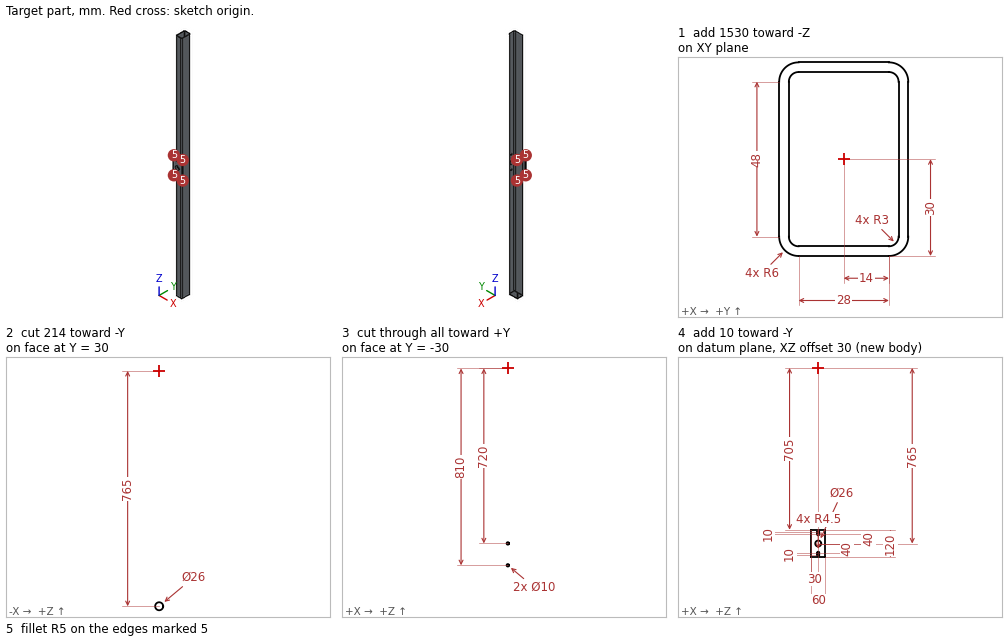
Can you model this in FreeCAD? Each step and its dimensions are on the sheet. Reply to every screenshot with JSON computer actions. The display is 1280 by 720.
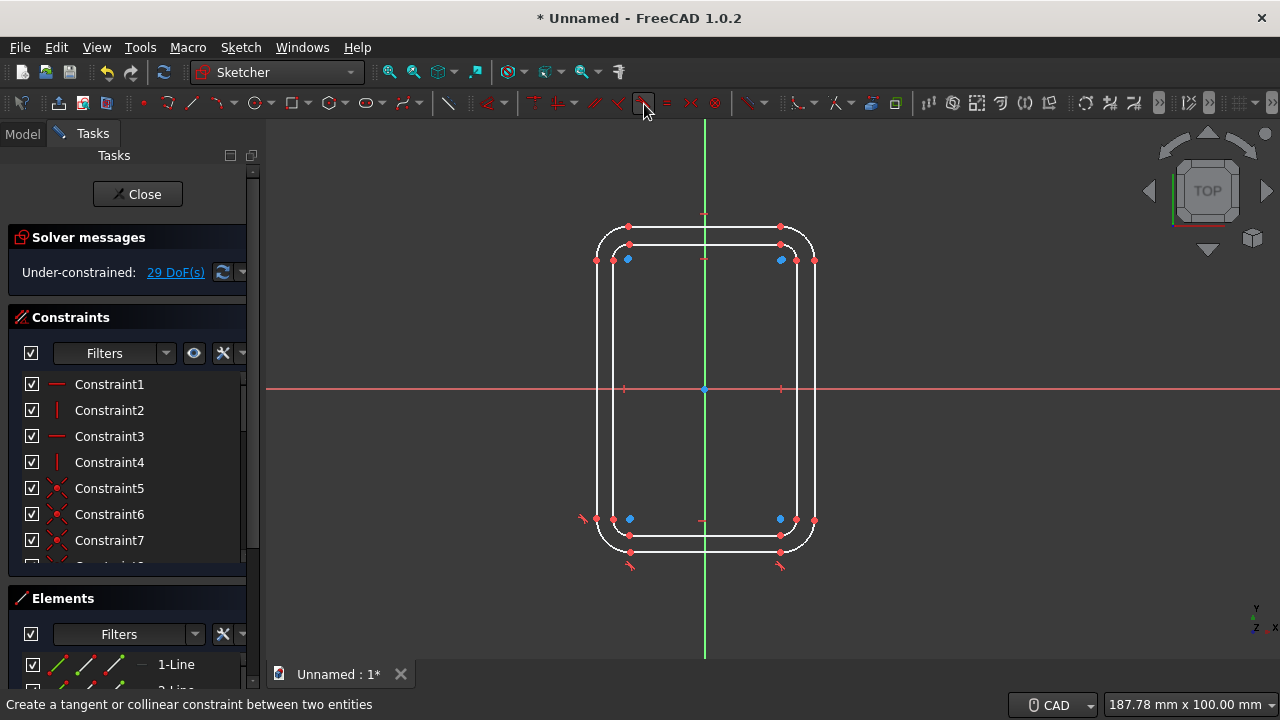
{"action": "left_click", "coordinate": [597, 441]}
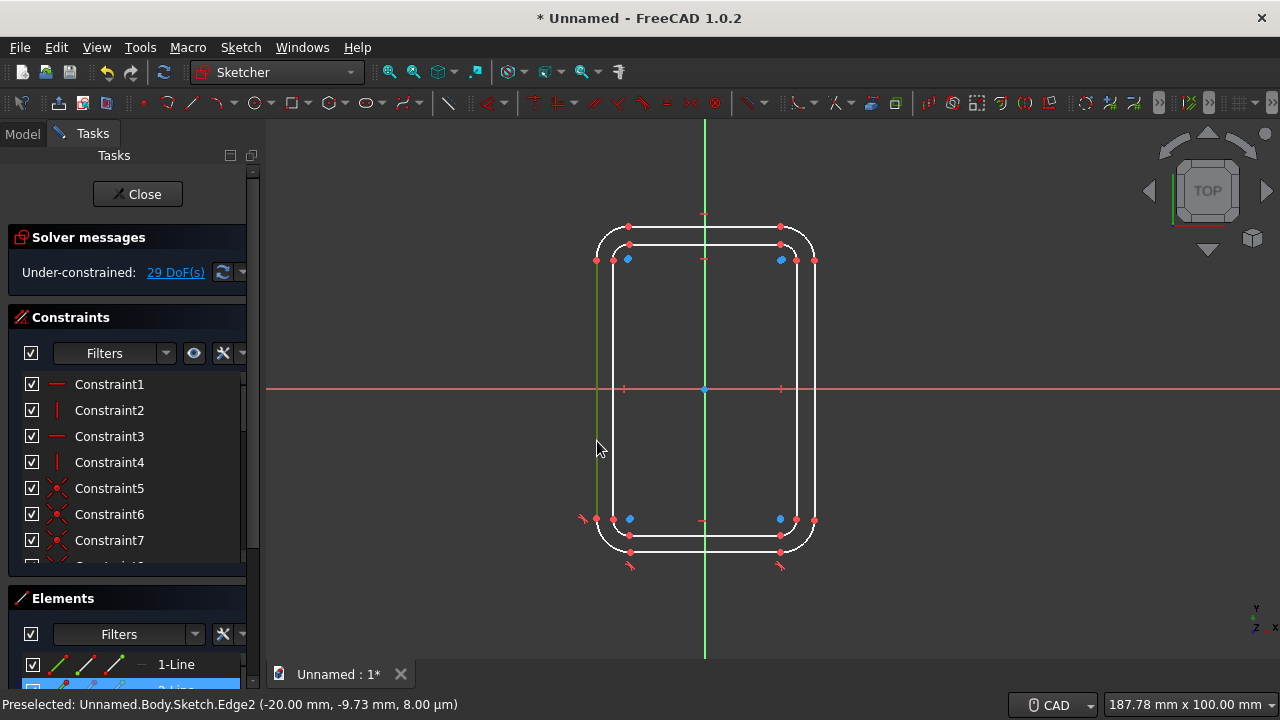
{"action": "left_click", "coordinate": [614, 230]}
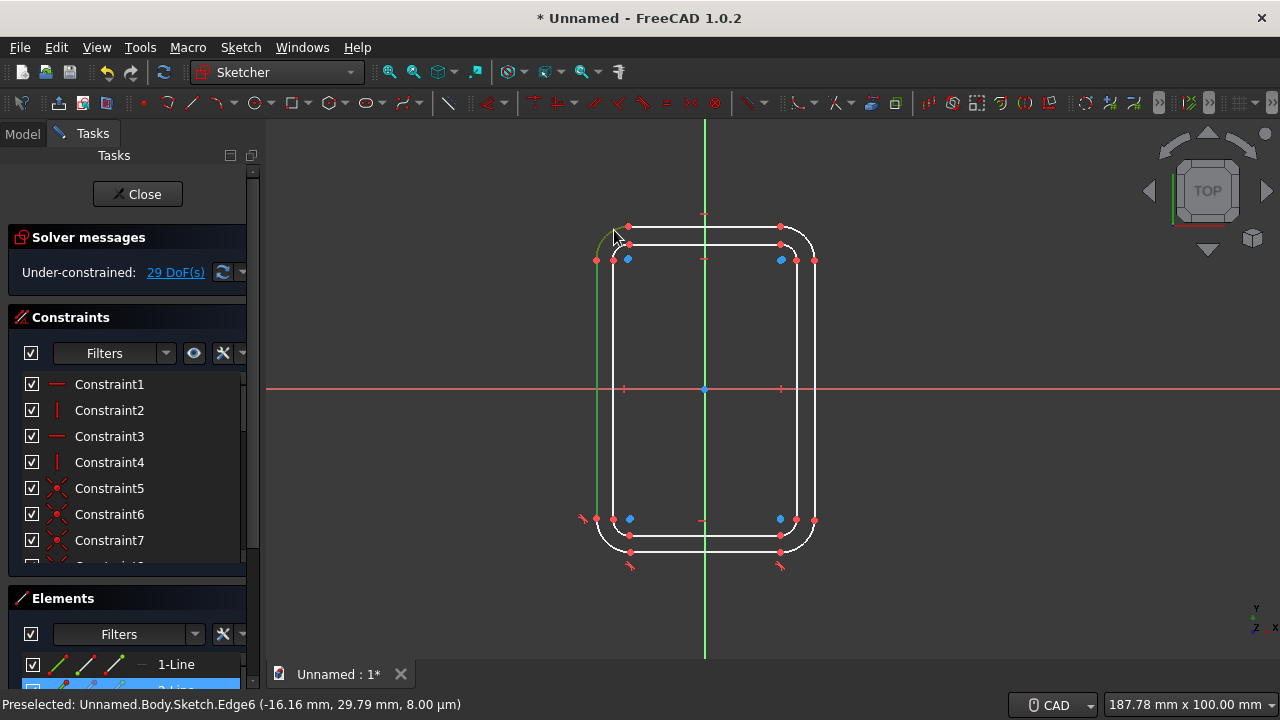
{"action": "left_click", "coordinate": [644, 104]}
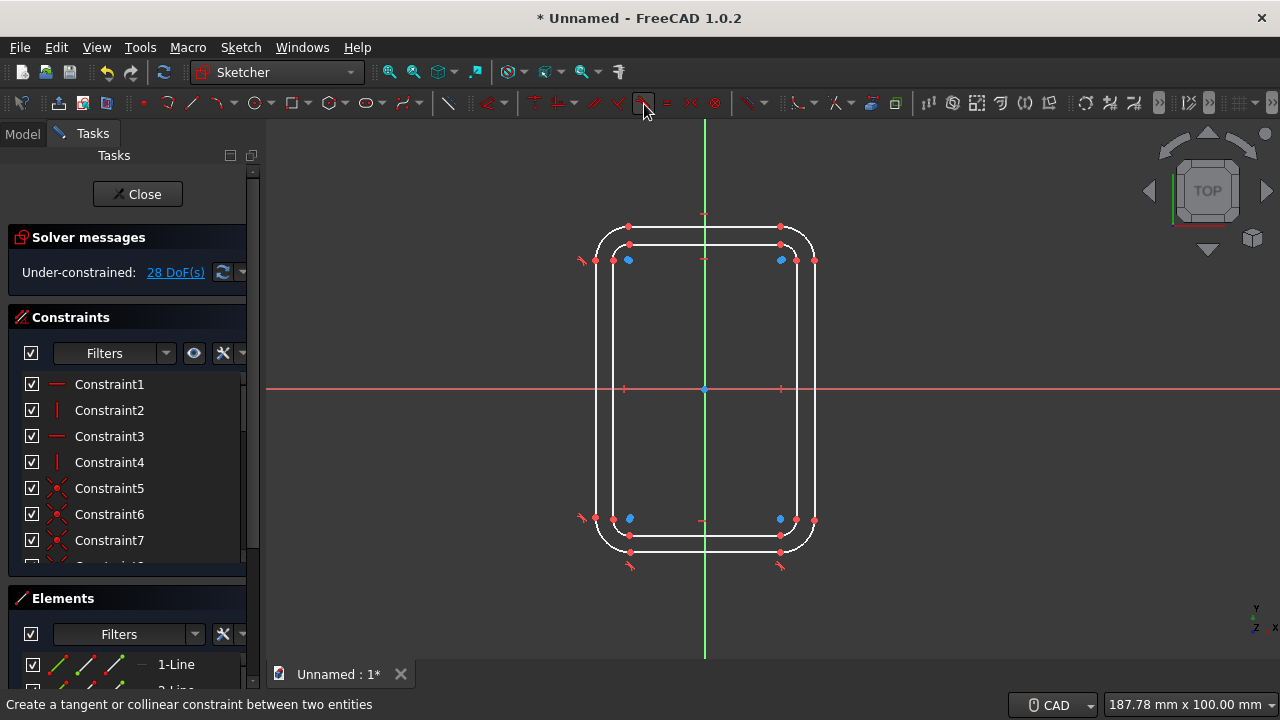
{"action": "left_click", "coordinate": [674, 227]}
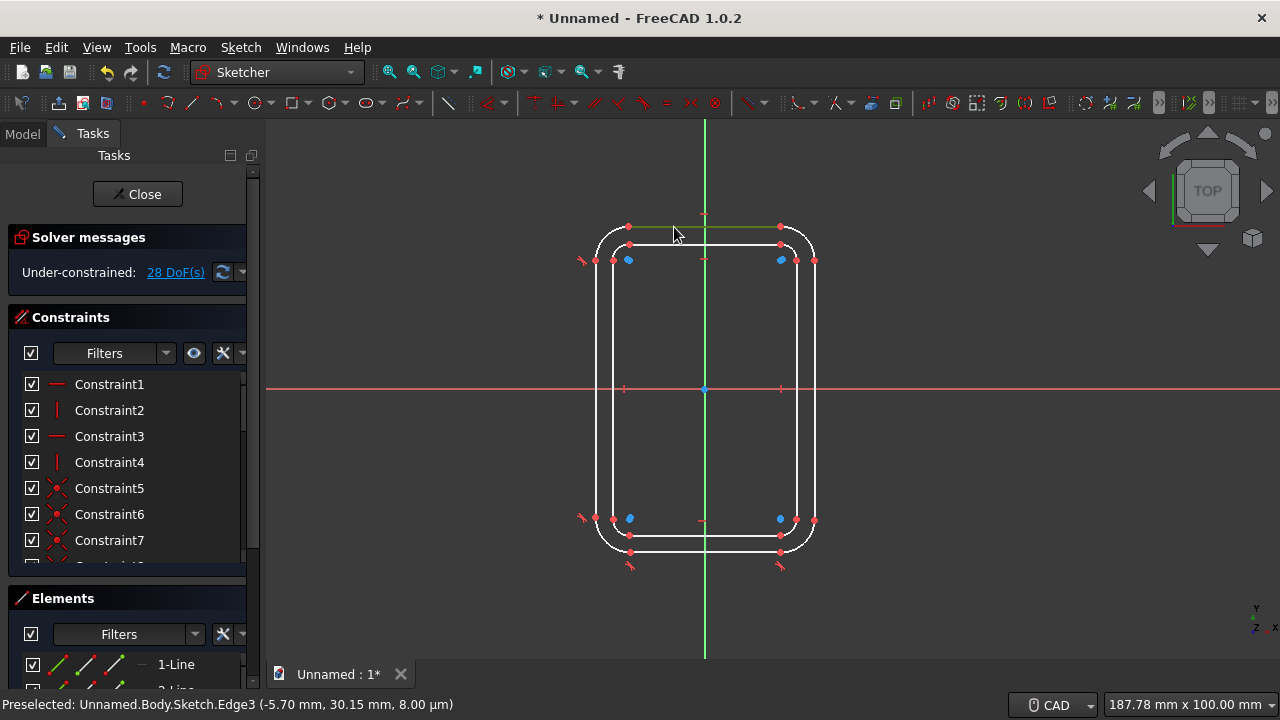
{"action": "left_click", "coordinate": [614, 231]}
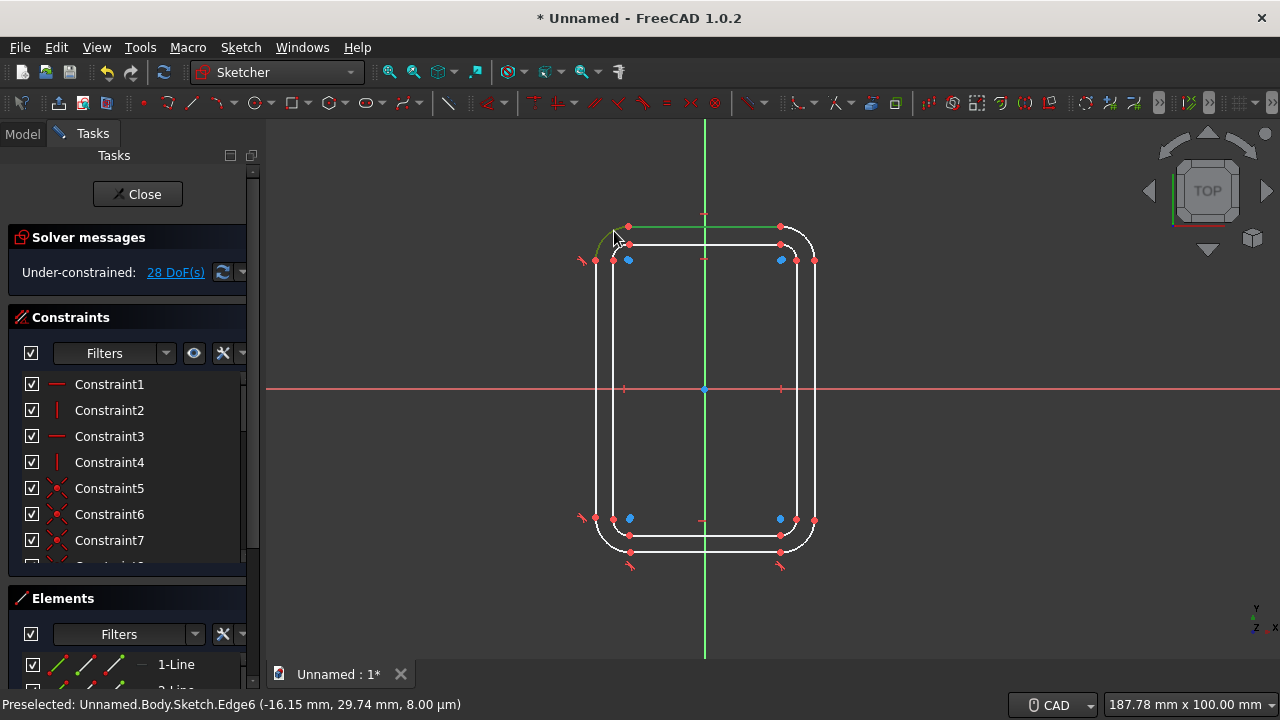
{"action": "left_click", "coordinate": [644, 104]}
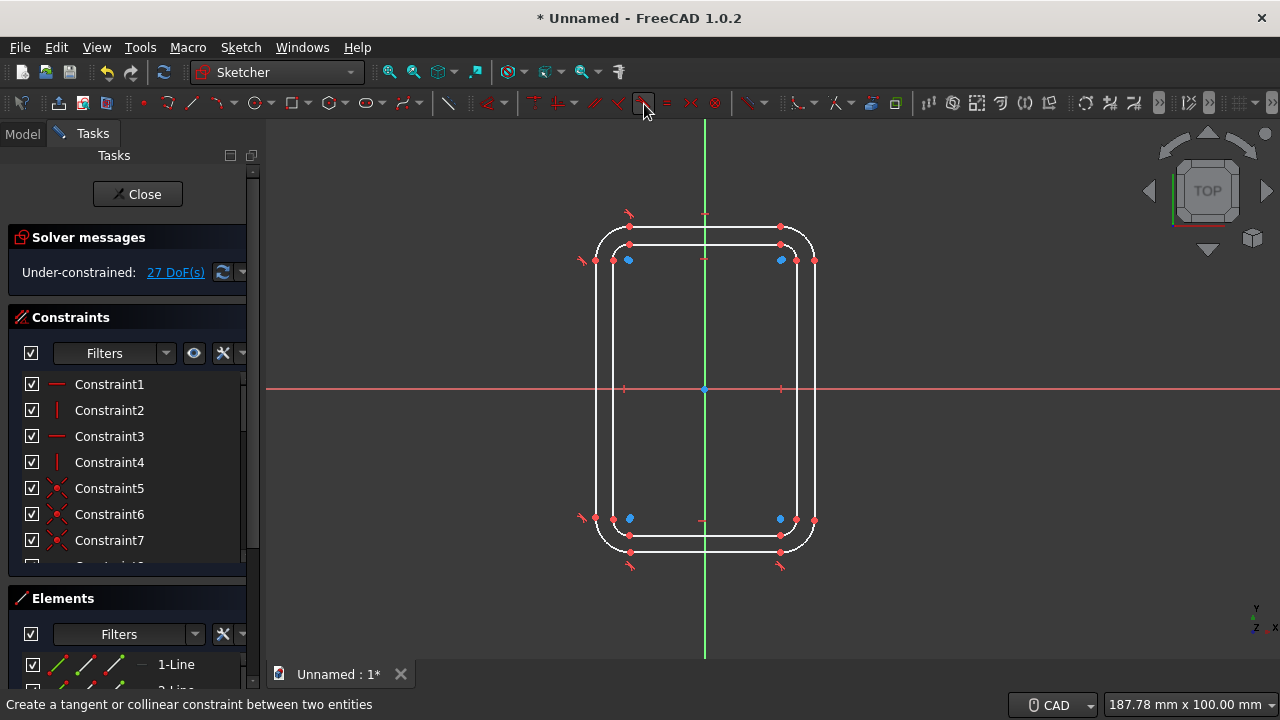
{"action": "left_click", "coordinate": [675, 227]}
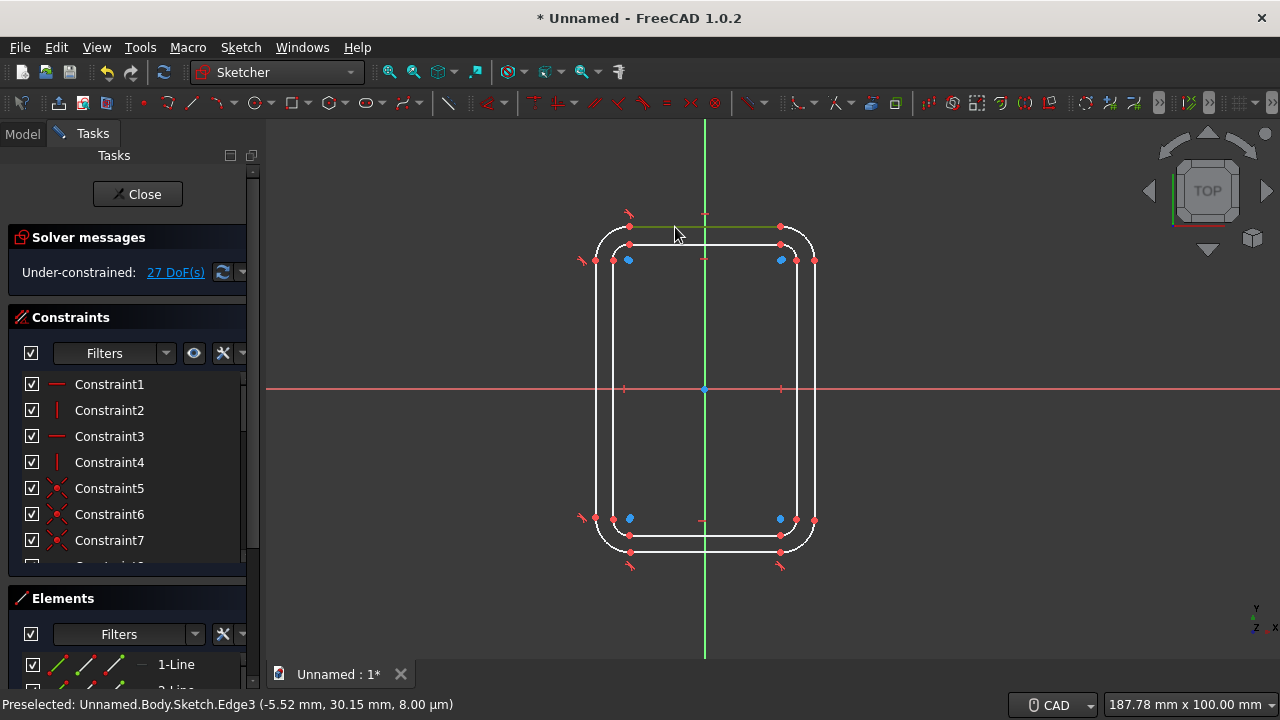
{"action": "left_click", "coordinate": [811, 245]}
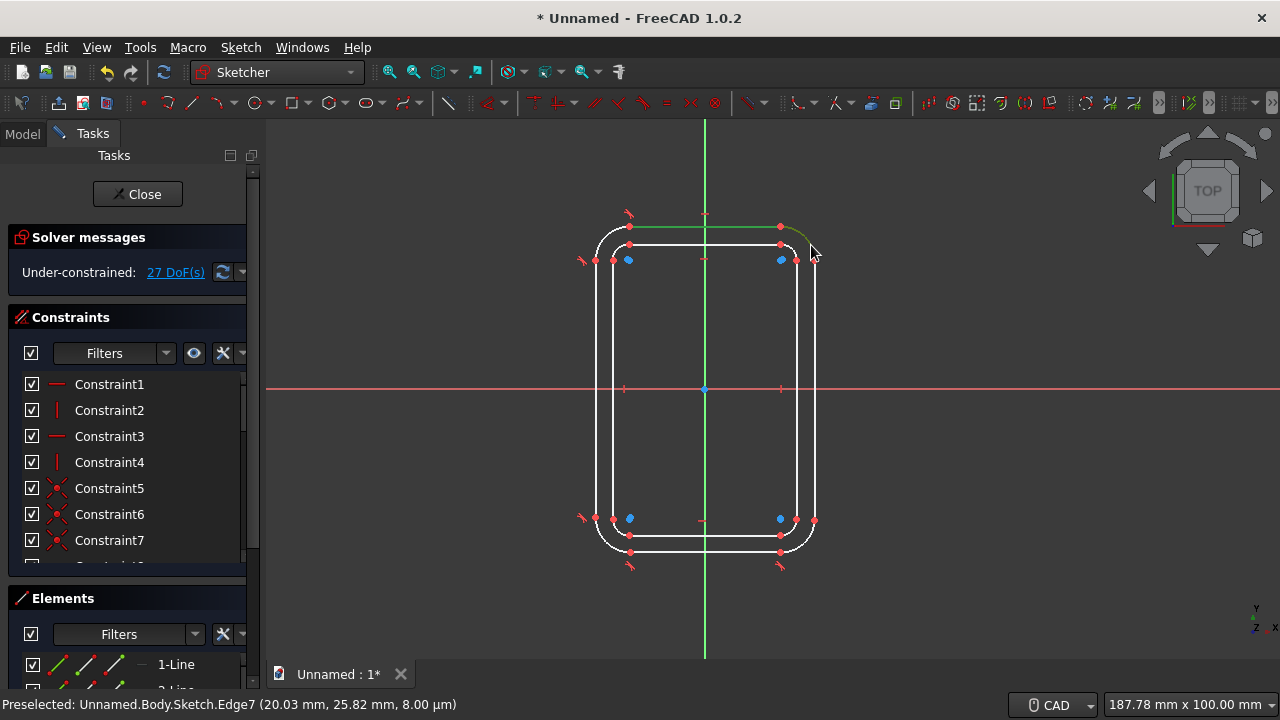
{"action": "left_click", "coordinate": [644, 104]}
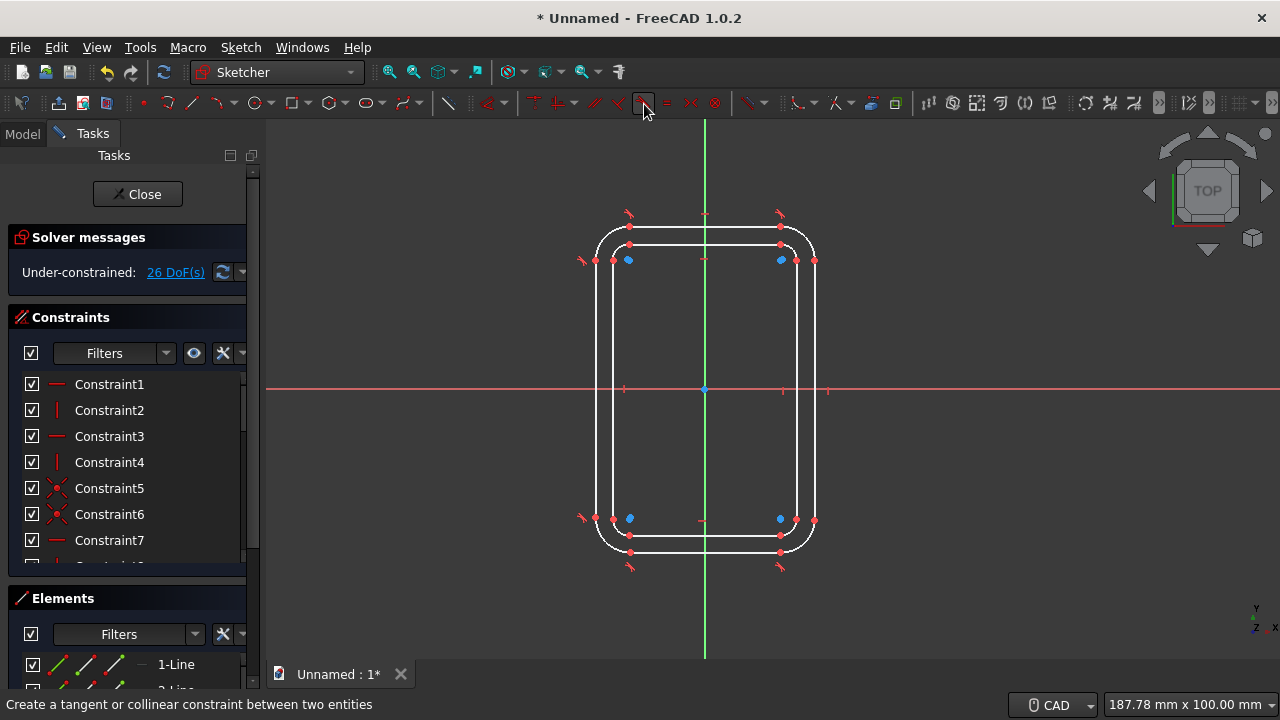
{"action": "left_click", "coordinate": [815, 338]}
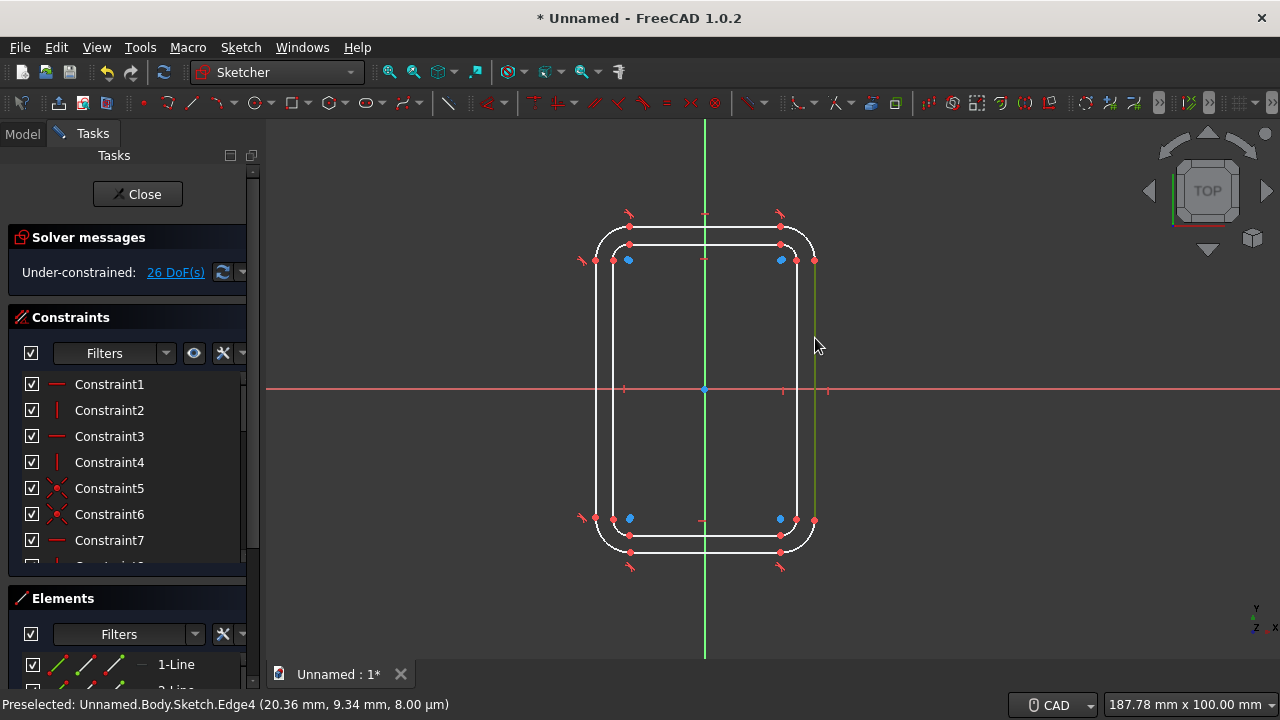
{"action": "left_click", "coordinate": [811, 245]}